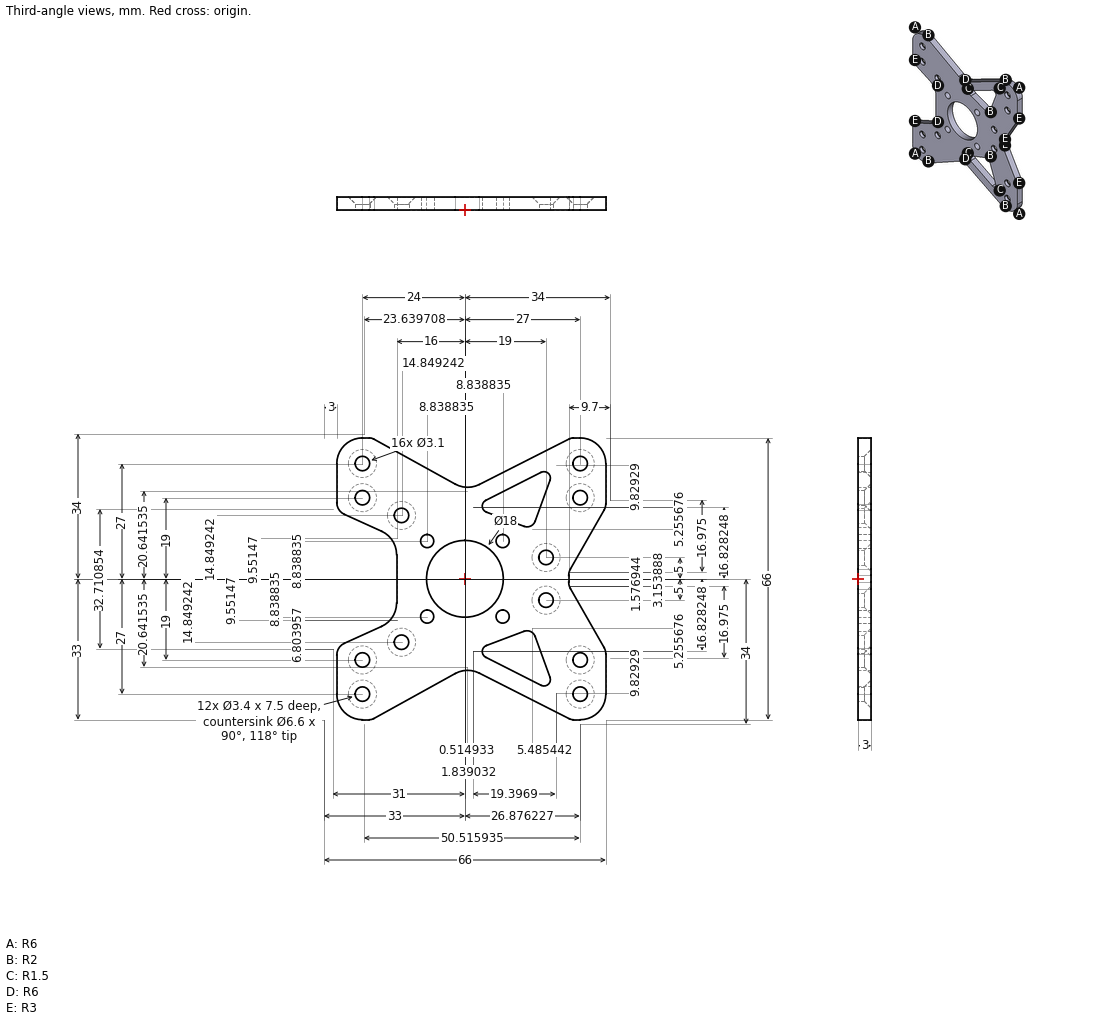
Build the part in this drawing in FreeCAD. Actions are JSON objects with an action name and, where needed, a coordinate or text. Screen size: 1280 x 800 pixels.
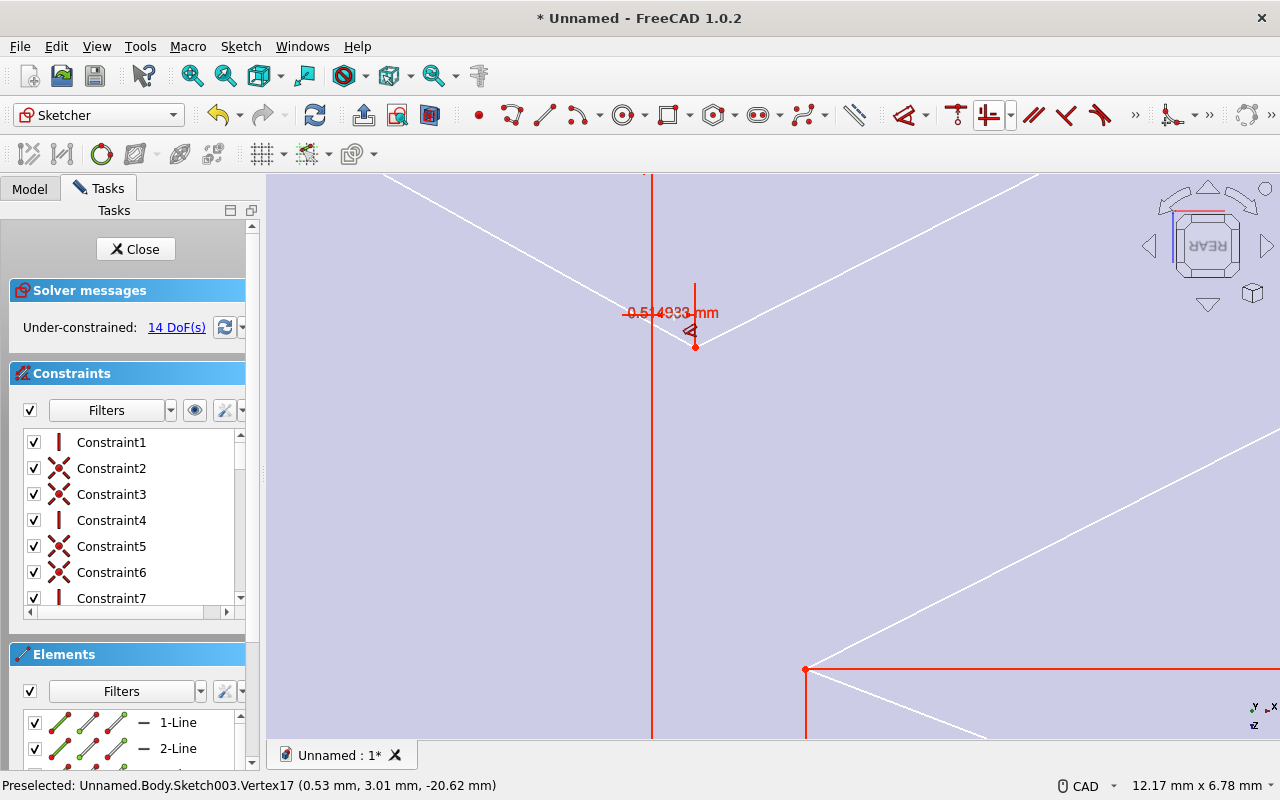
{"action": "scroll", "coordinate": [700, 352], "scroll_direction": "down", "scroll_amount": 14}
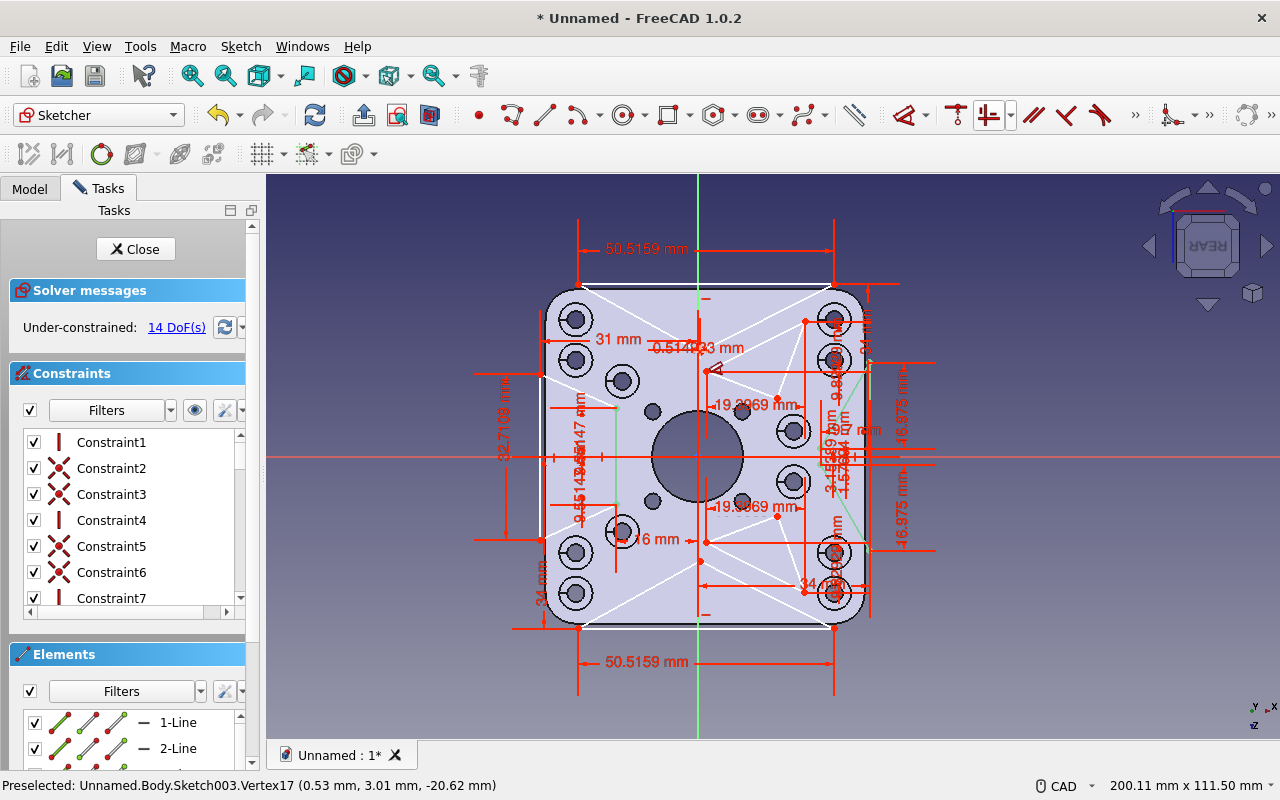
{"action": "scroll", "coordinate": [707, 372], "scroll_direction": "up", "scroll_amount": 8}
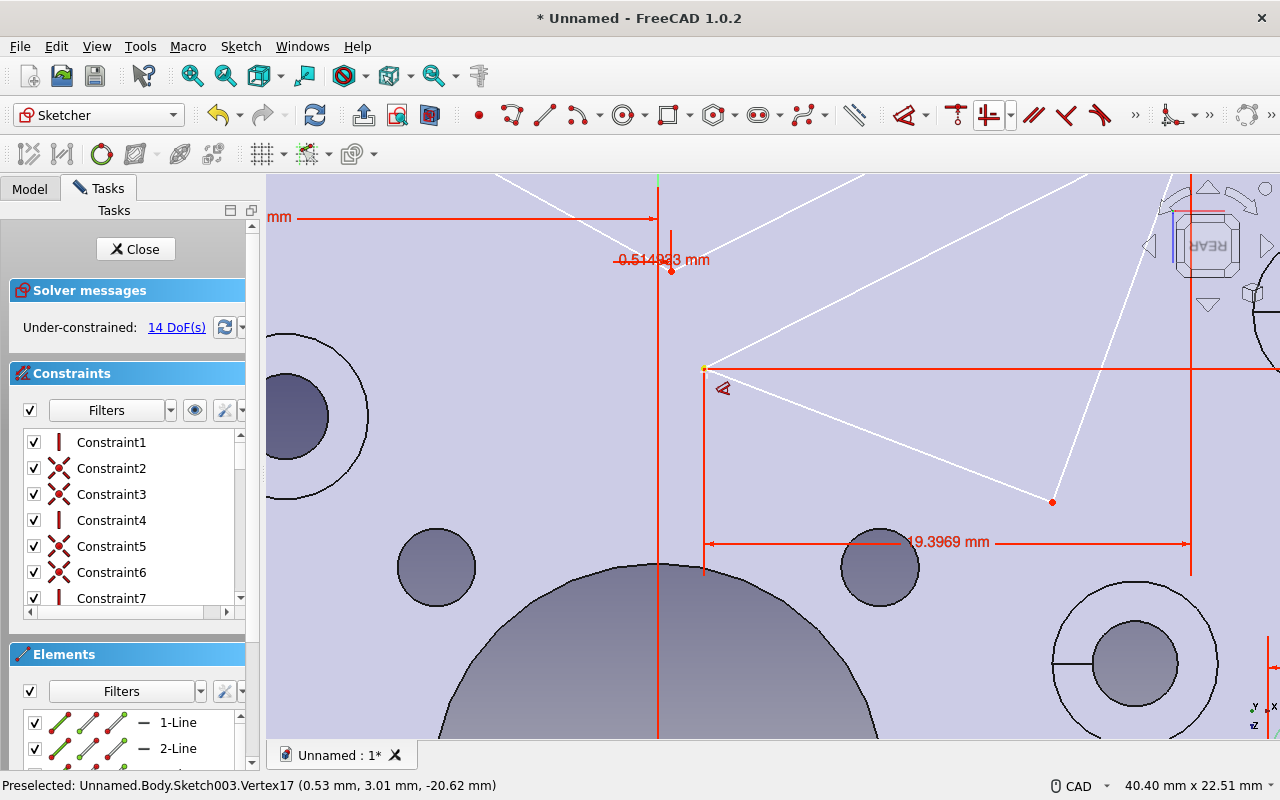
{"action": "left_click", "coordinate": [704, 369]}
{"action": "left_click", "coordinate": [681, 335]}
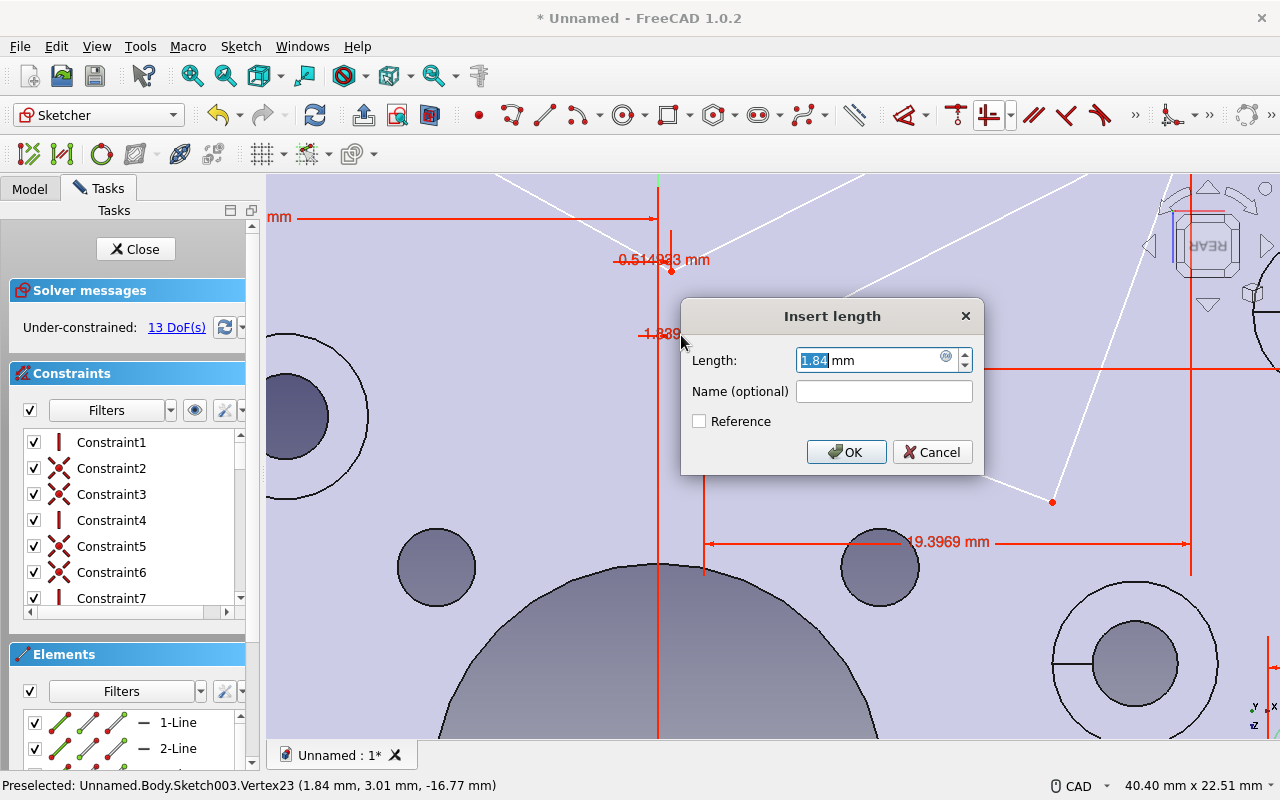
{"action": "type", "text": "1.839032"}
{"action": "key", "text": "Return"}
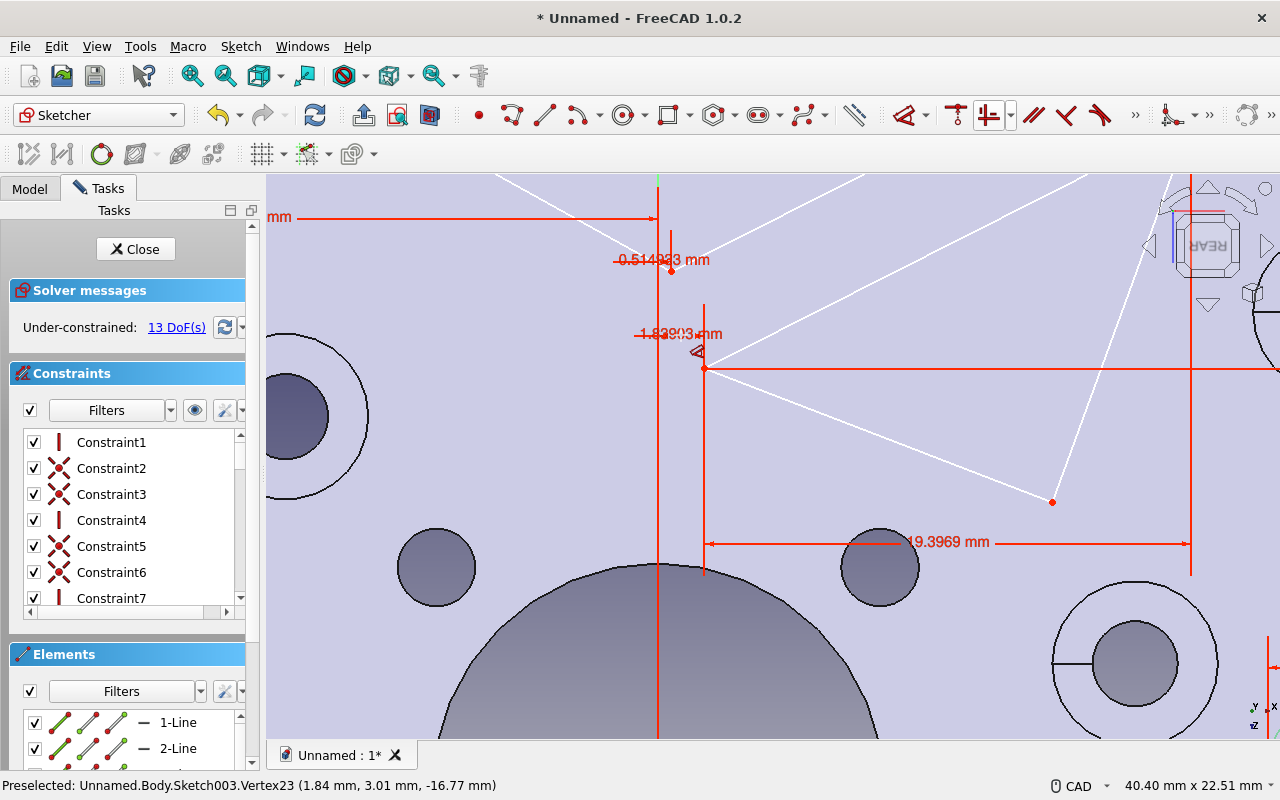
{"action": "scroll", "coordinate": [707, 372], "scroll_direction": "down", "scroll_amount": 8}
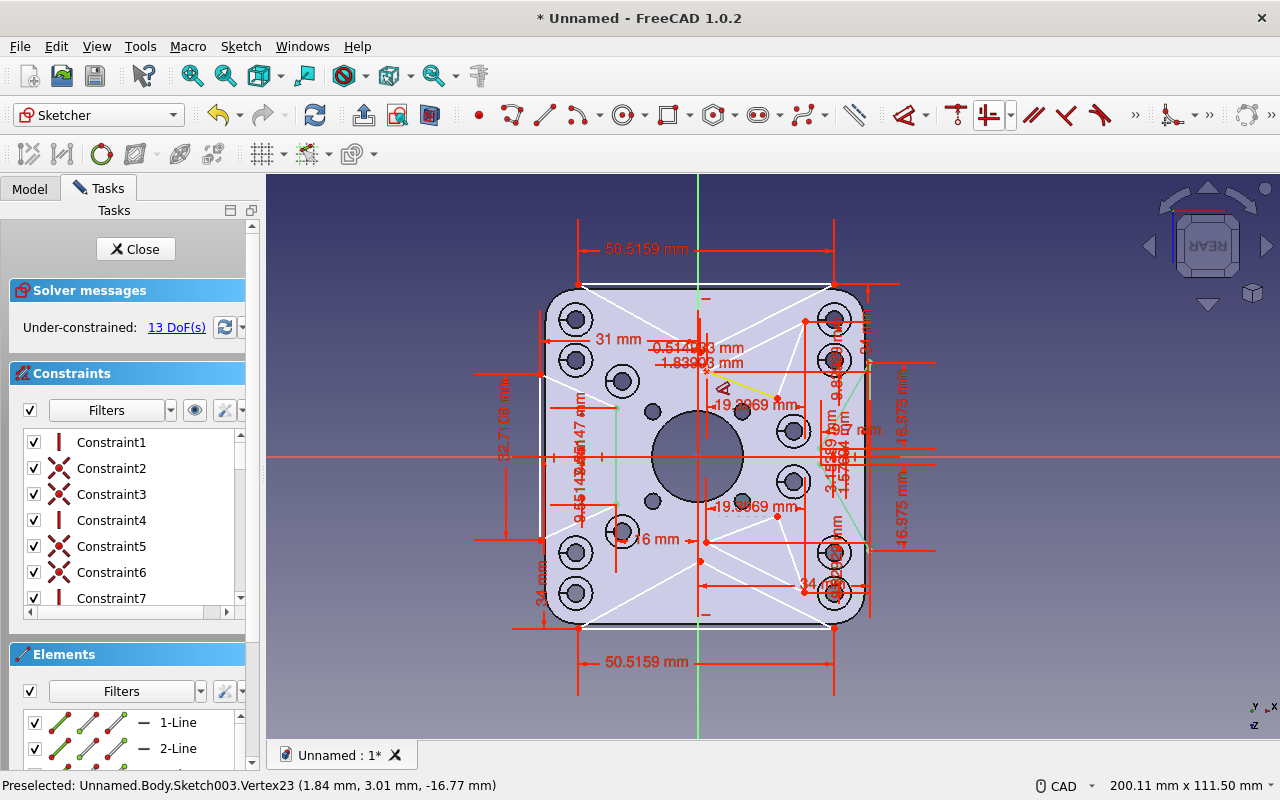
{"action": "scroll", "coordinate": [706, 543], "scroll_direction": "up", "scroll_amount": 8}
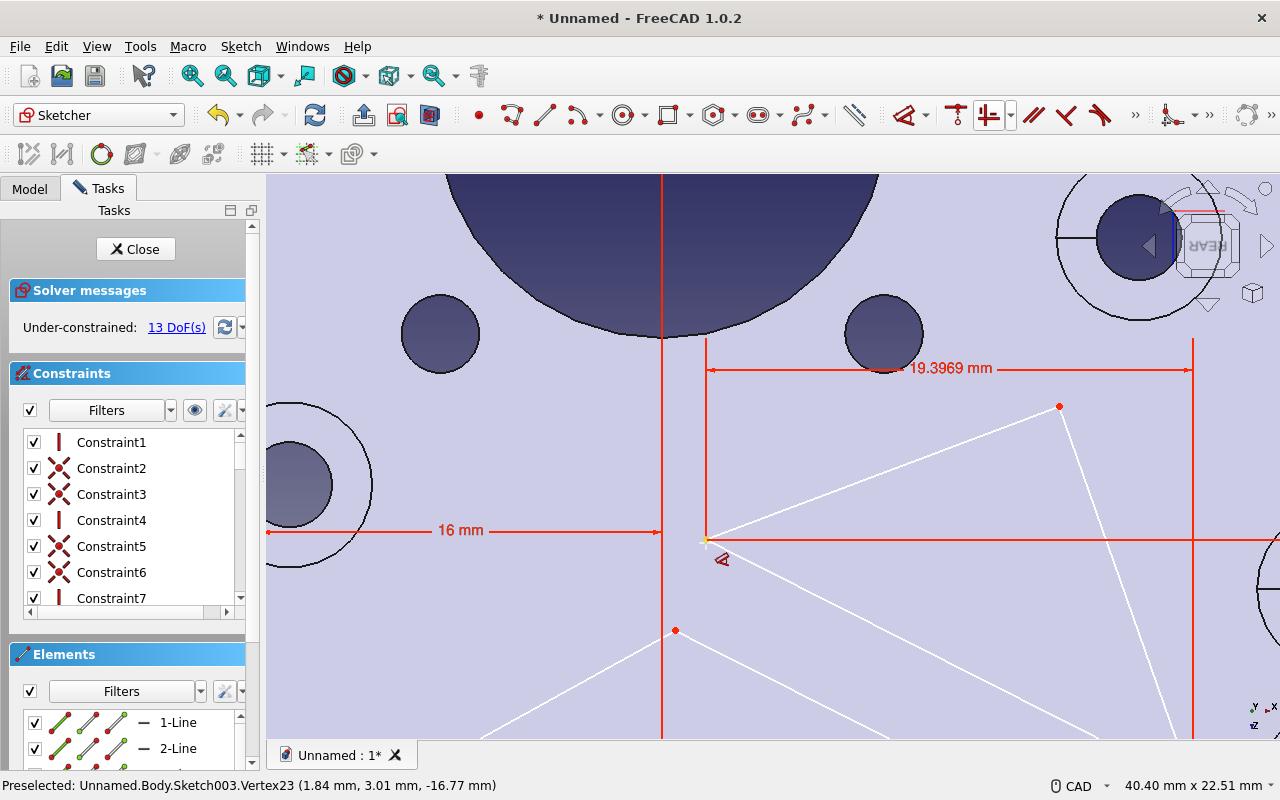
{"action": "left_click", "coordinate": [706, 540]}
{"action": "left_click", "coordinate": [684, 574]}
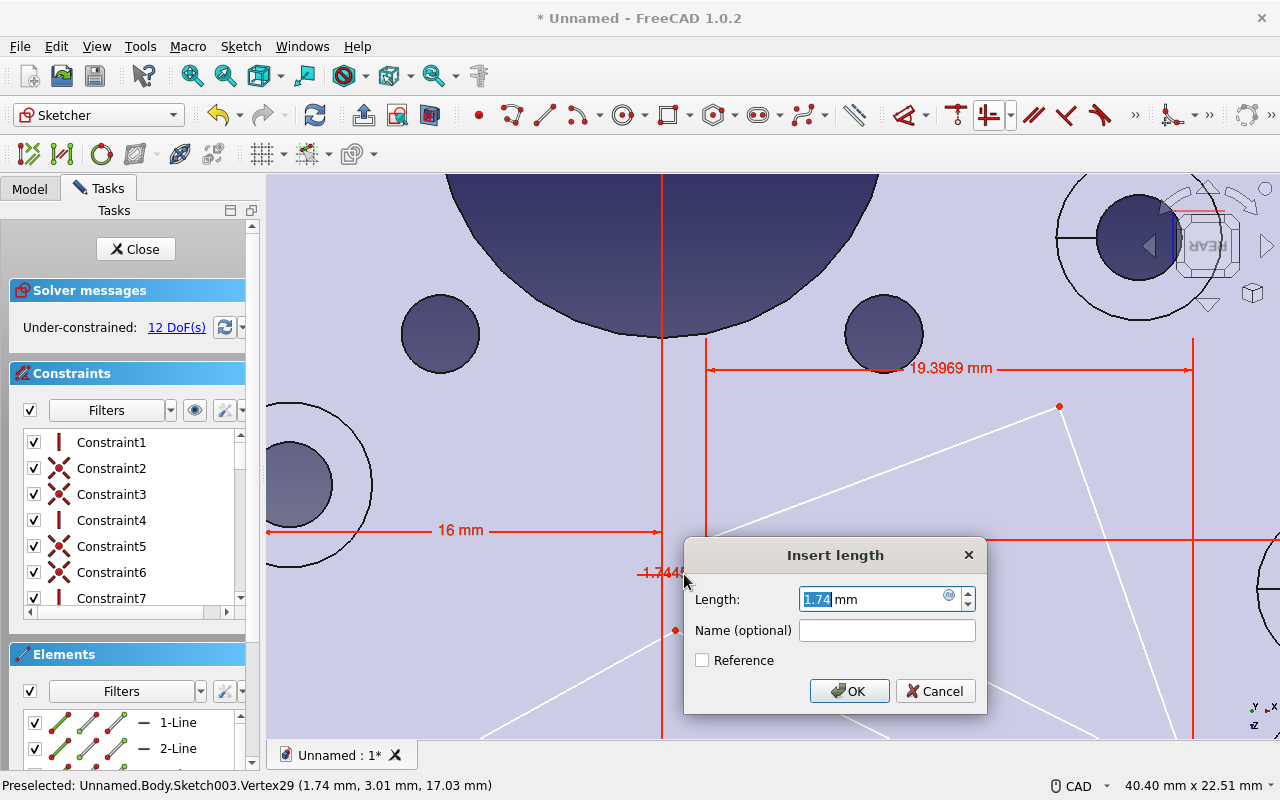
{"action": "type", "text": "1.839032"}
{"action": "key", "text": "Return"}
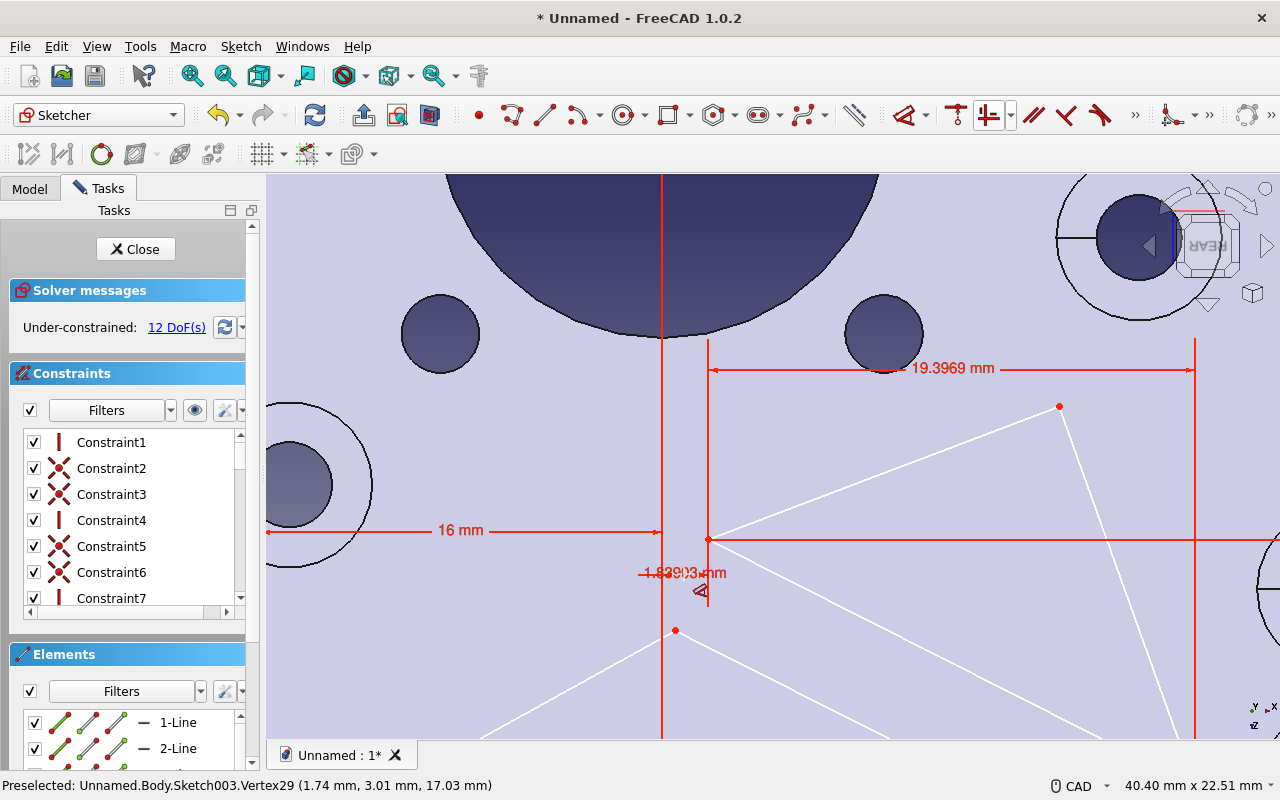
{"action": "scroll", "coordinate": [675, 631], "scroll_direction": "up", "scroll_amount": 6}